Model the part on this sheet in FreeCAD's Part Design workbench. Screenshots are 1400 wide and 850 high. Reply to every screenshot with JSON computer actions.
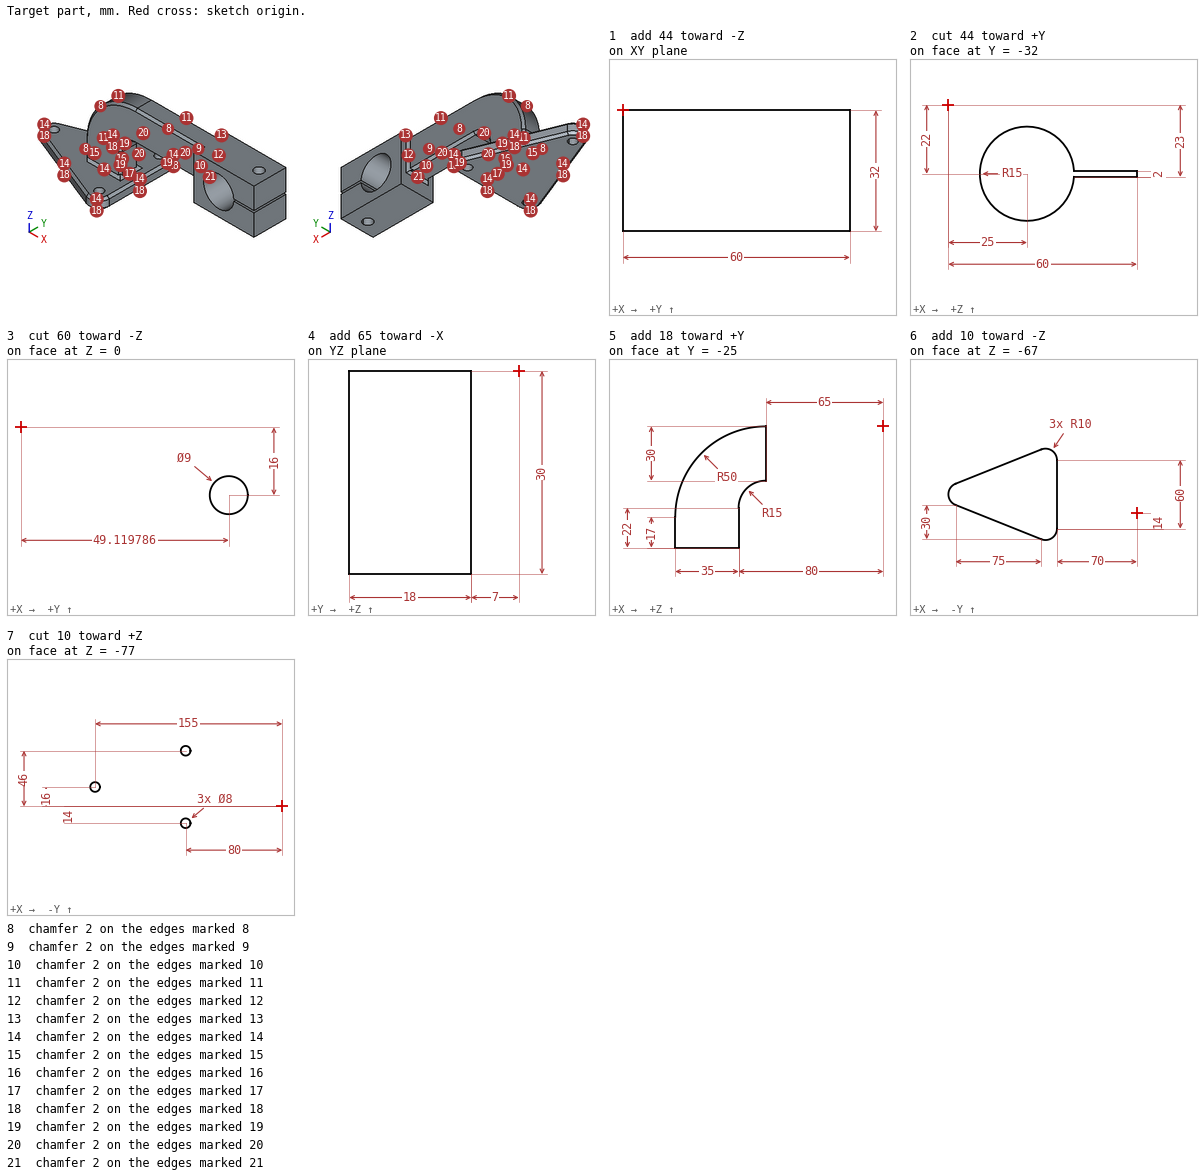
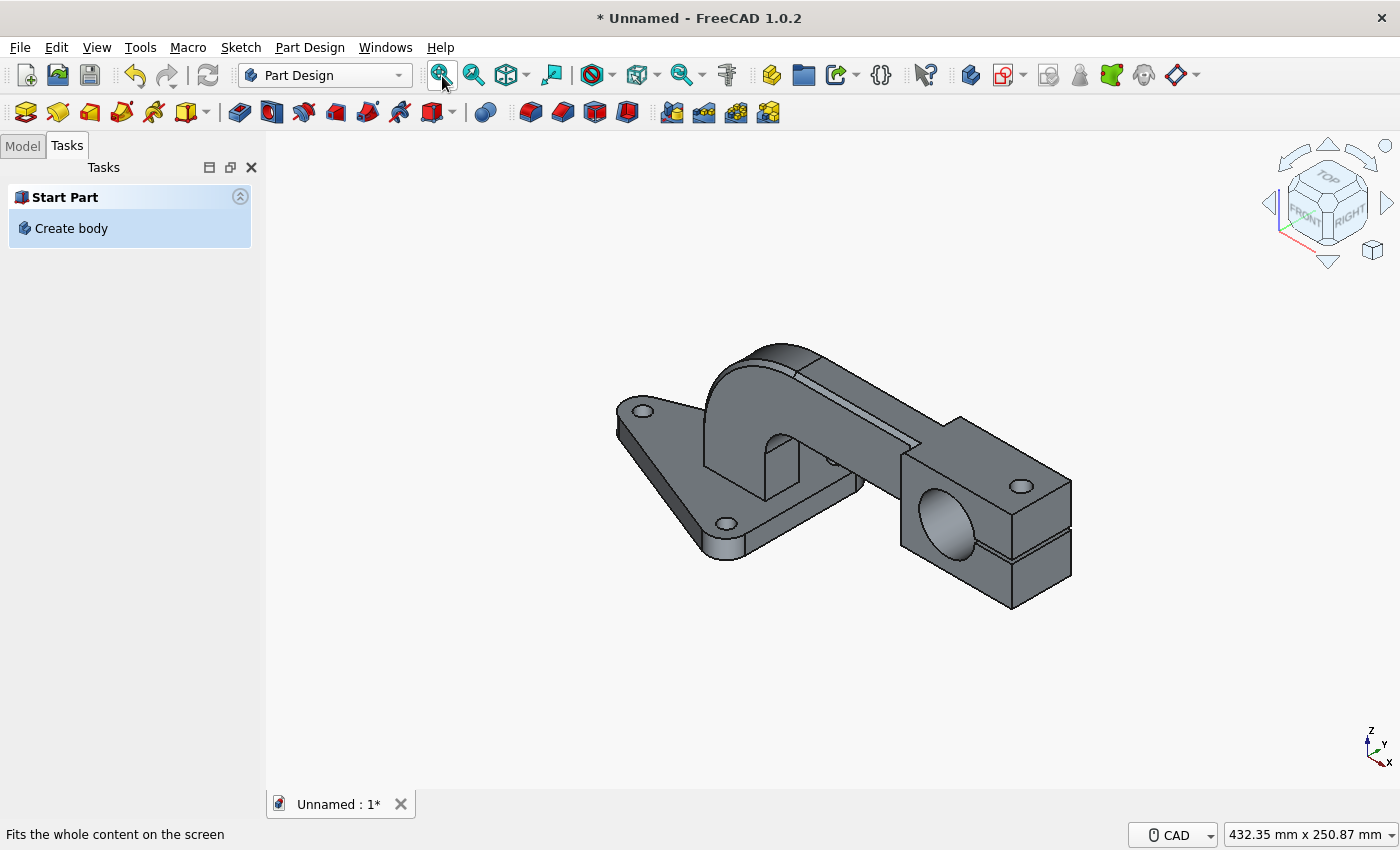
{"action": "key", "text": "2"}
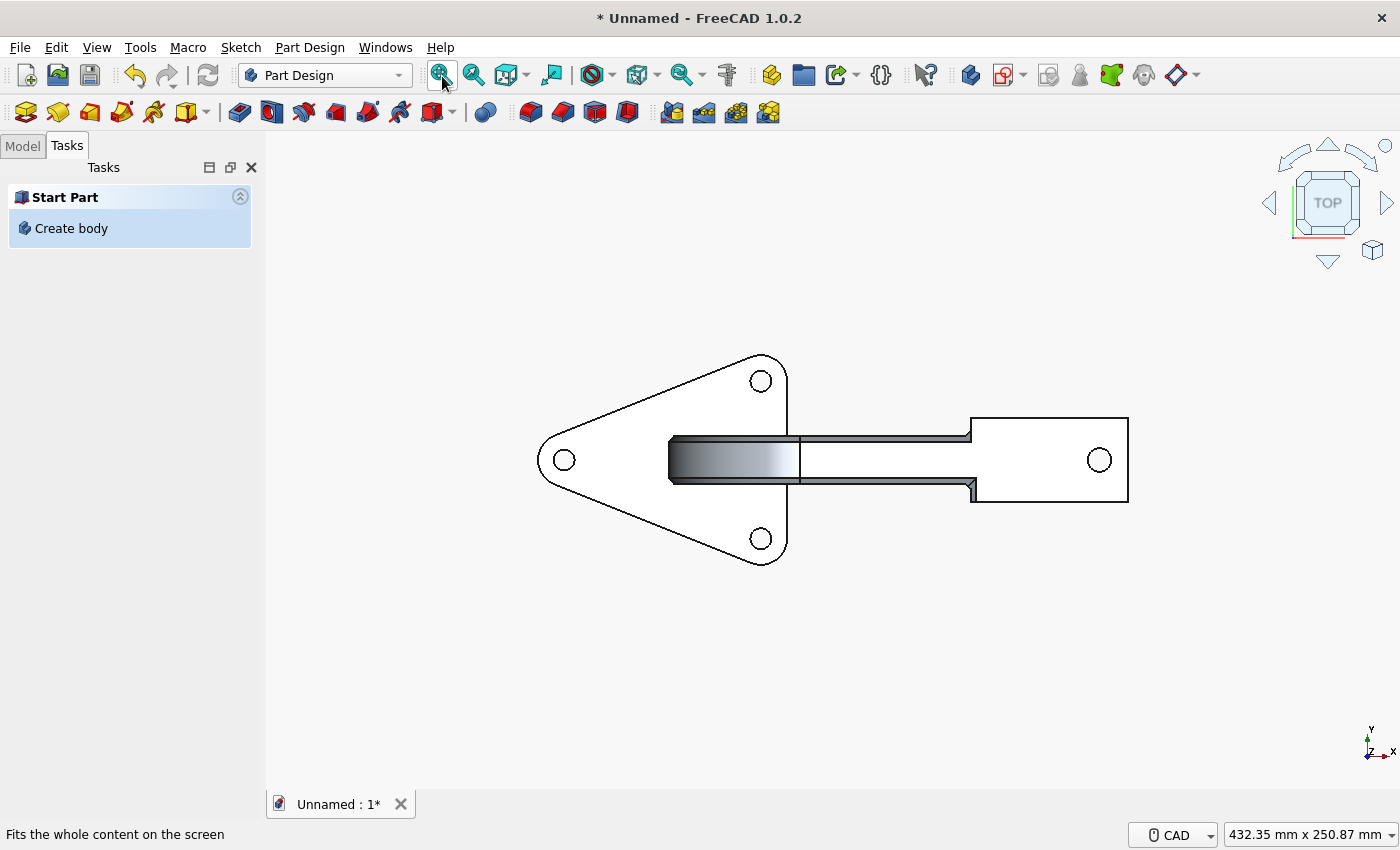
{"action": "left_click", "coordinate": [971, 426]}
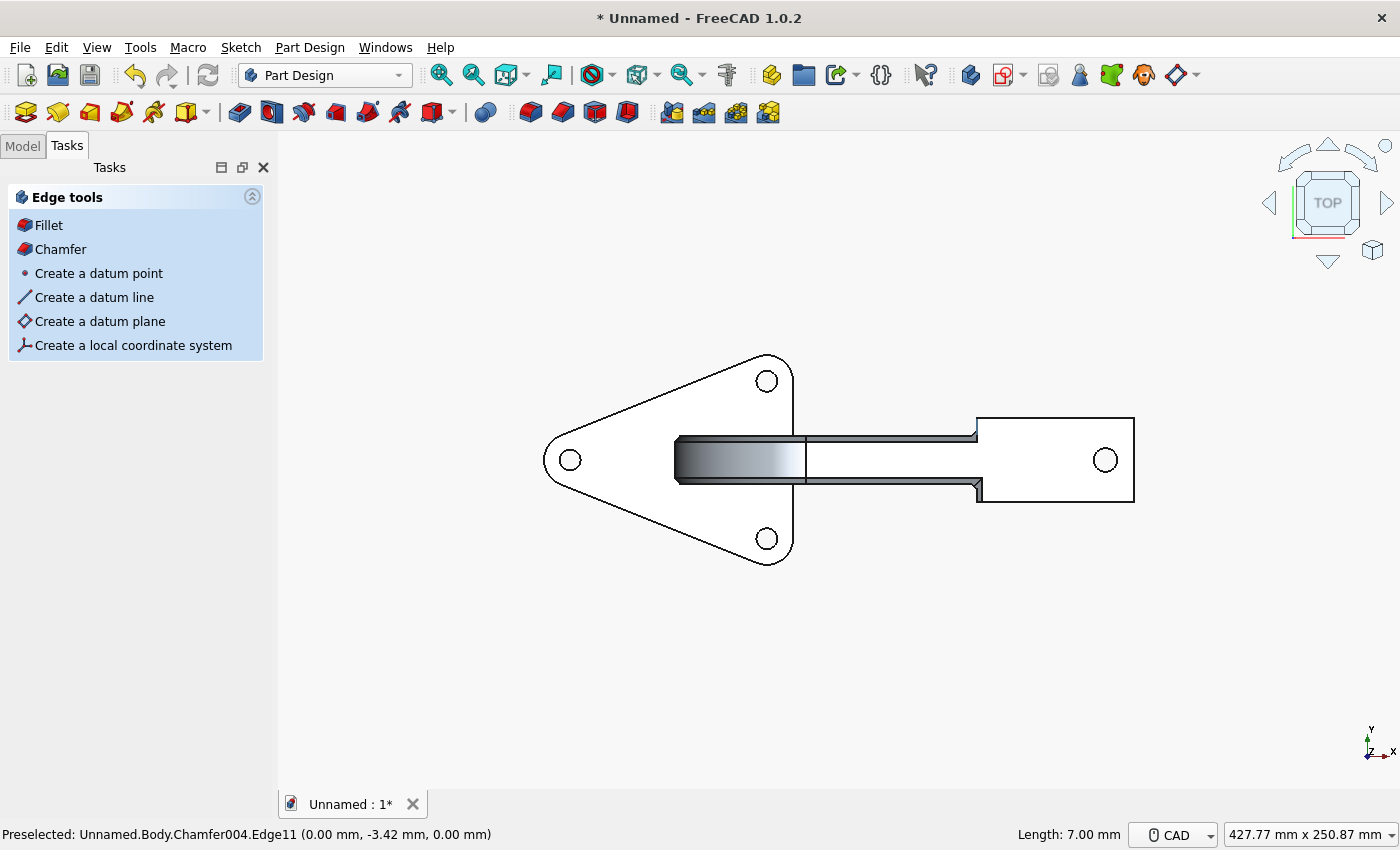
{"action": "left_click", "coordinate": [564, 112]}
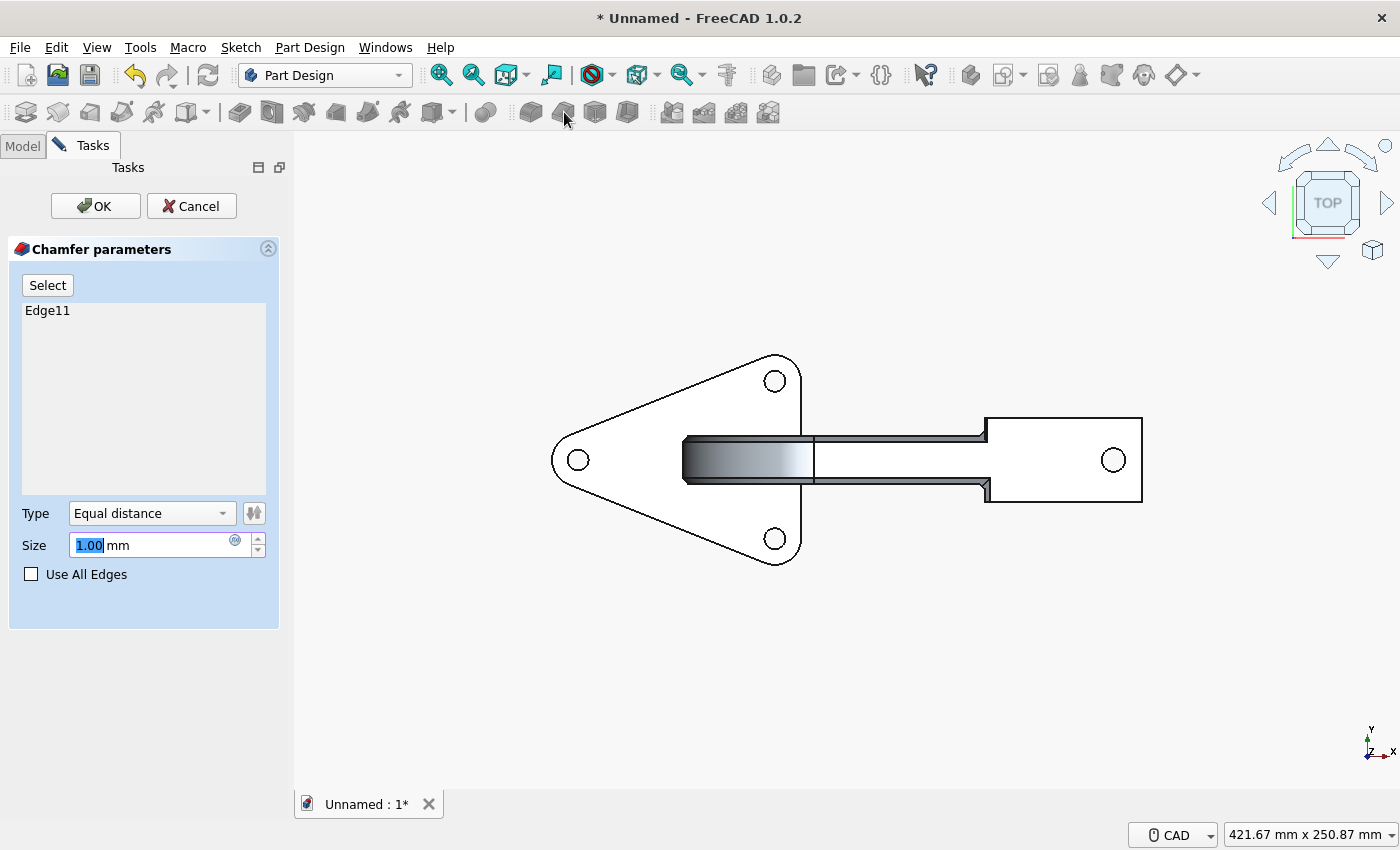
{"action": "type", "text": "2"}
{"action": "key", "text": "Tab"}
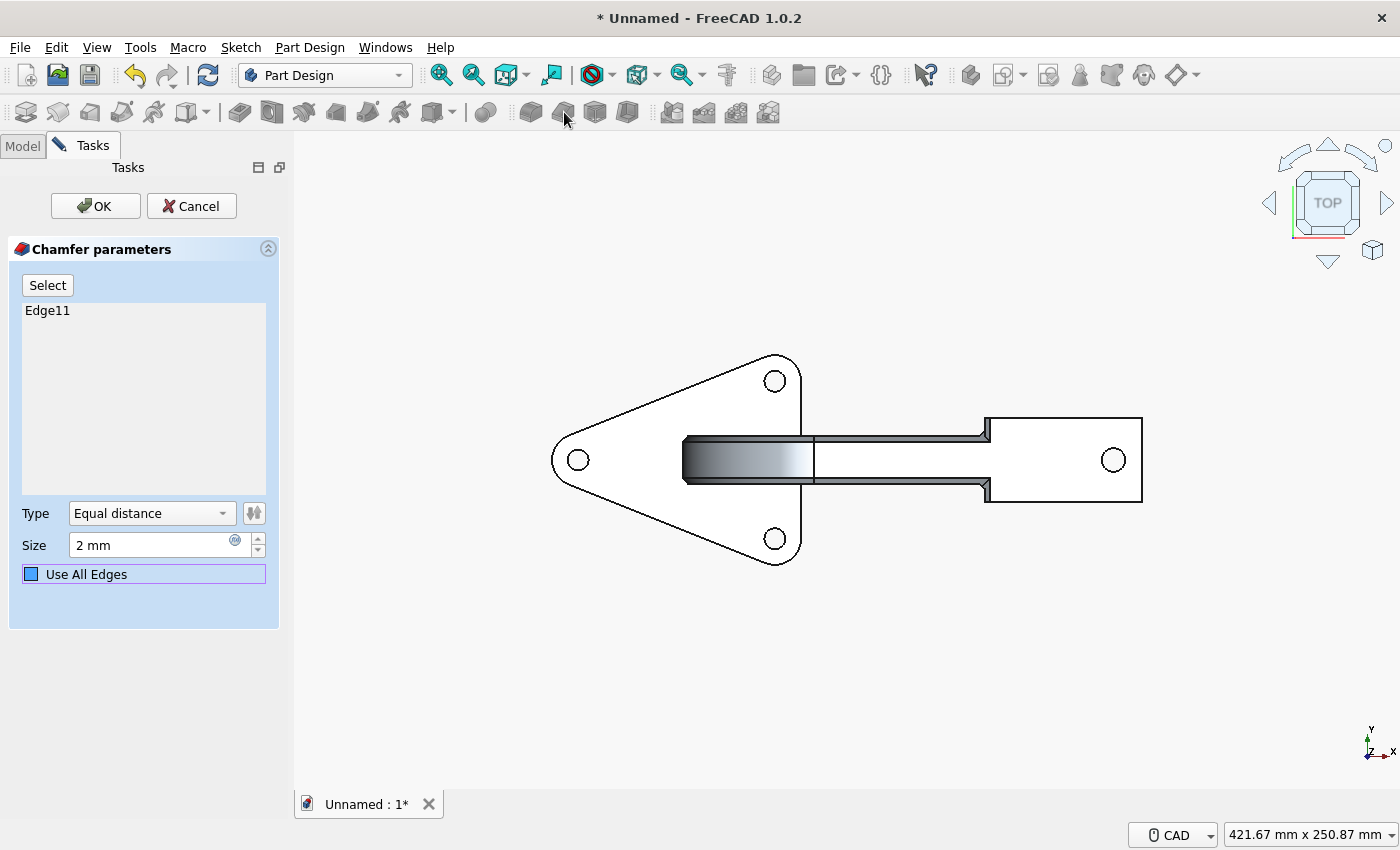
{"action": "left_click", "coordinate": [96, 206]}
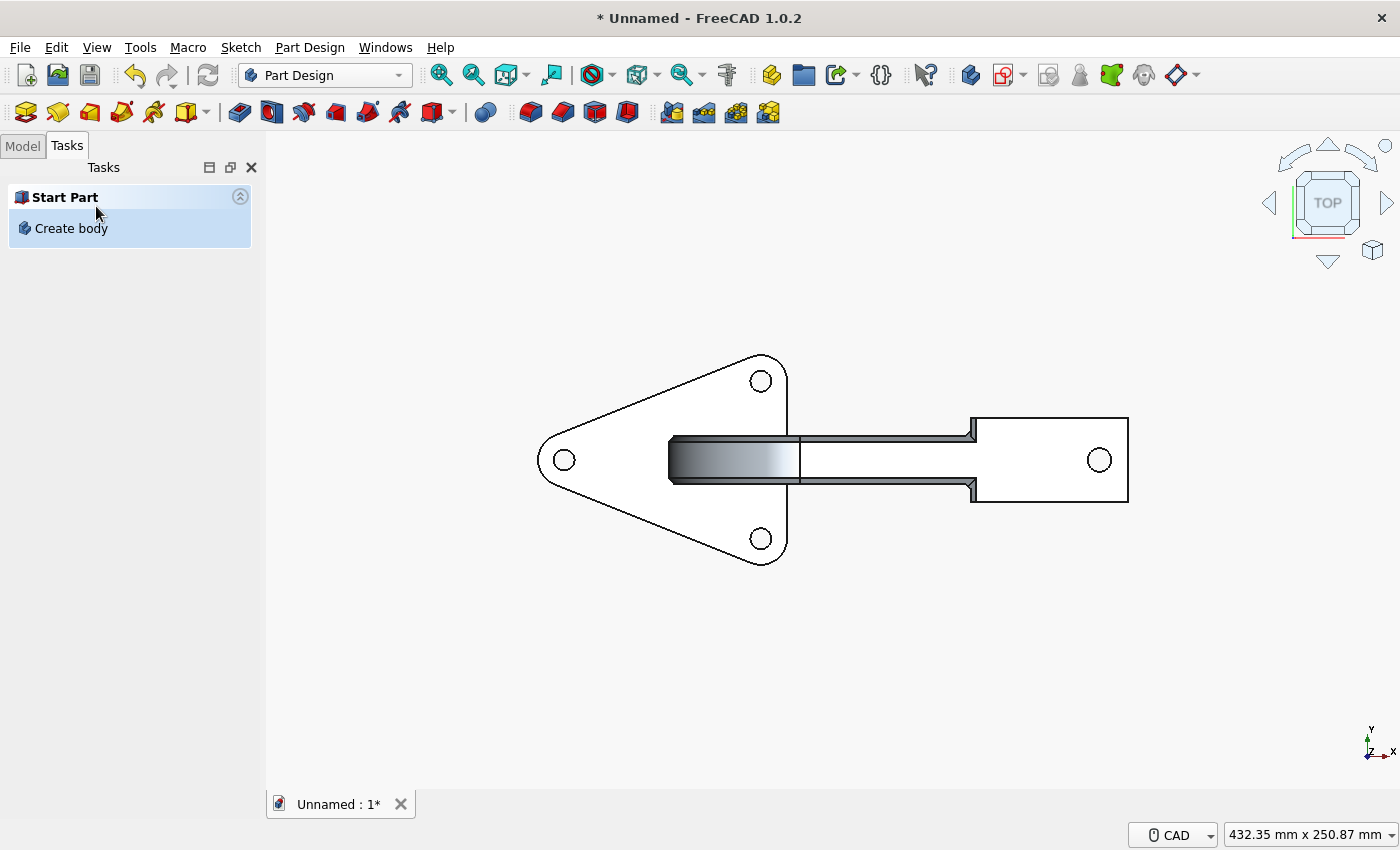
{"action": "left_click", "coordinate": [776, 359]}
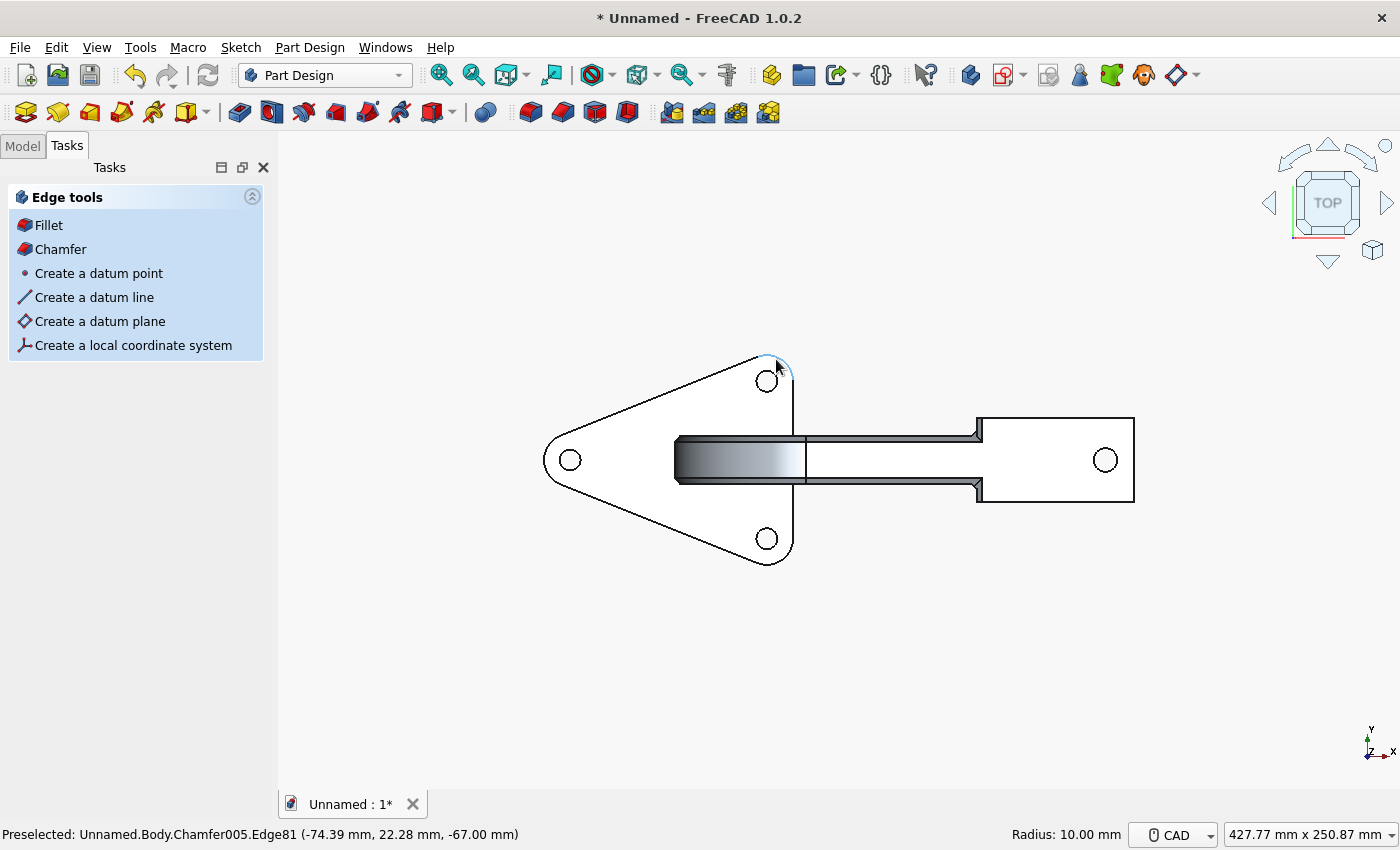
{"action": "left_click", "coordinate": [793, 428], "text": "ctrl"}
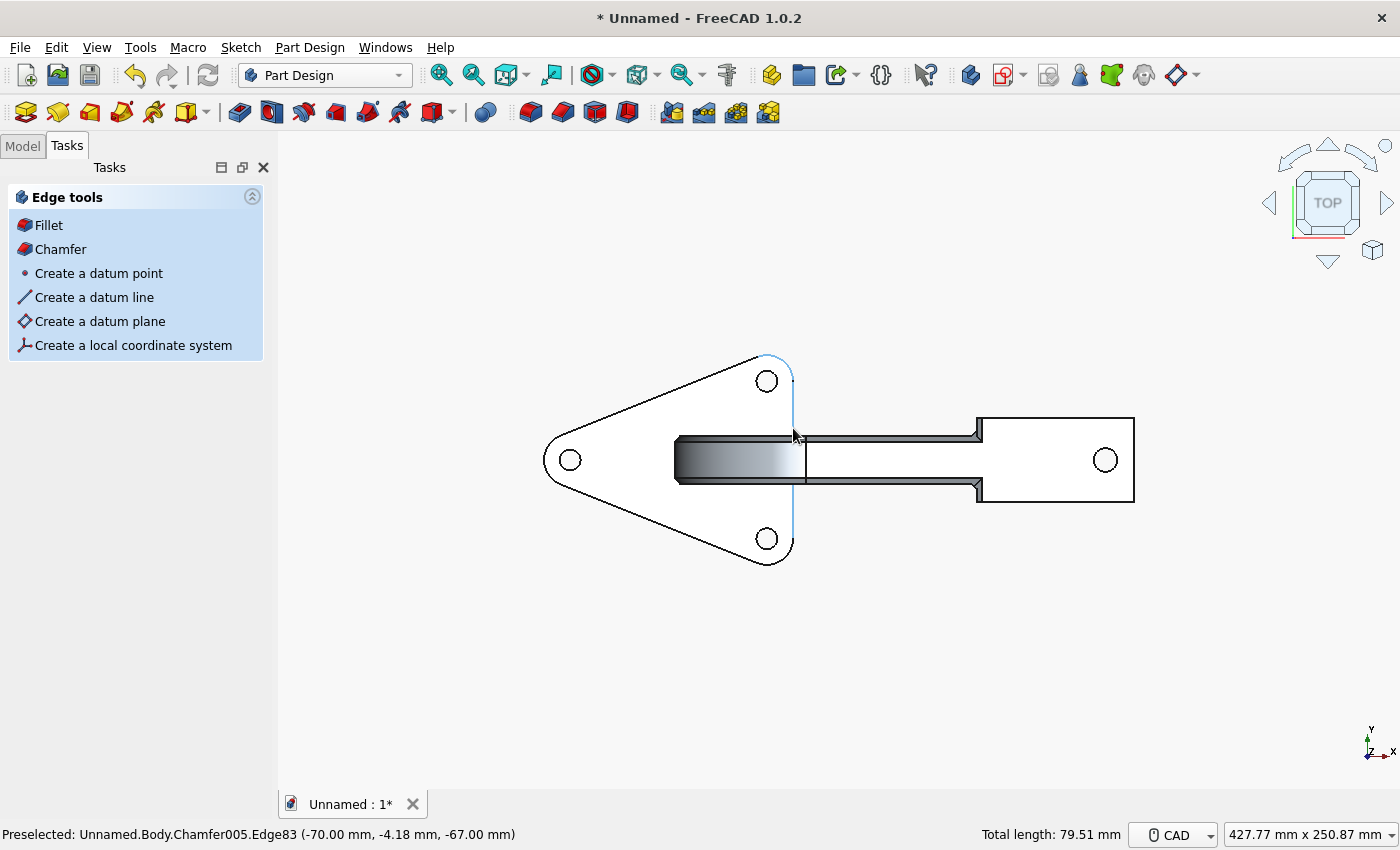
{"action": "left_click", "coordinate": [782, 559], "text": "ctrl"}